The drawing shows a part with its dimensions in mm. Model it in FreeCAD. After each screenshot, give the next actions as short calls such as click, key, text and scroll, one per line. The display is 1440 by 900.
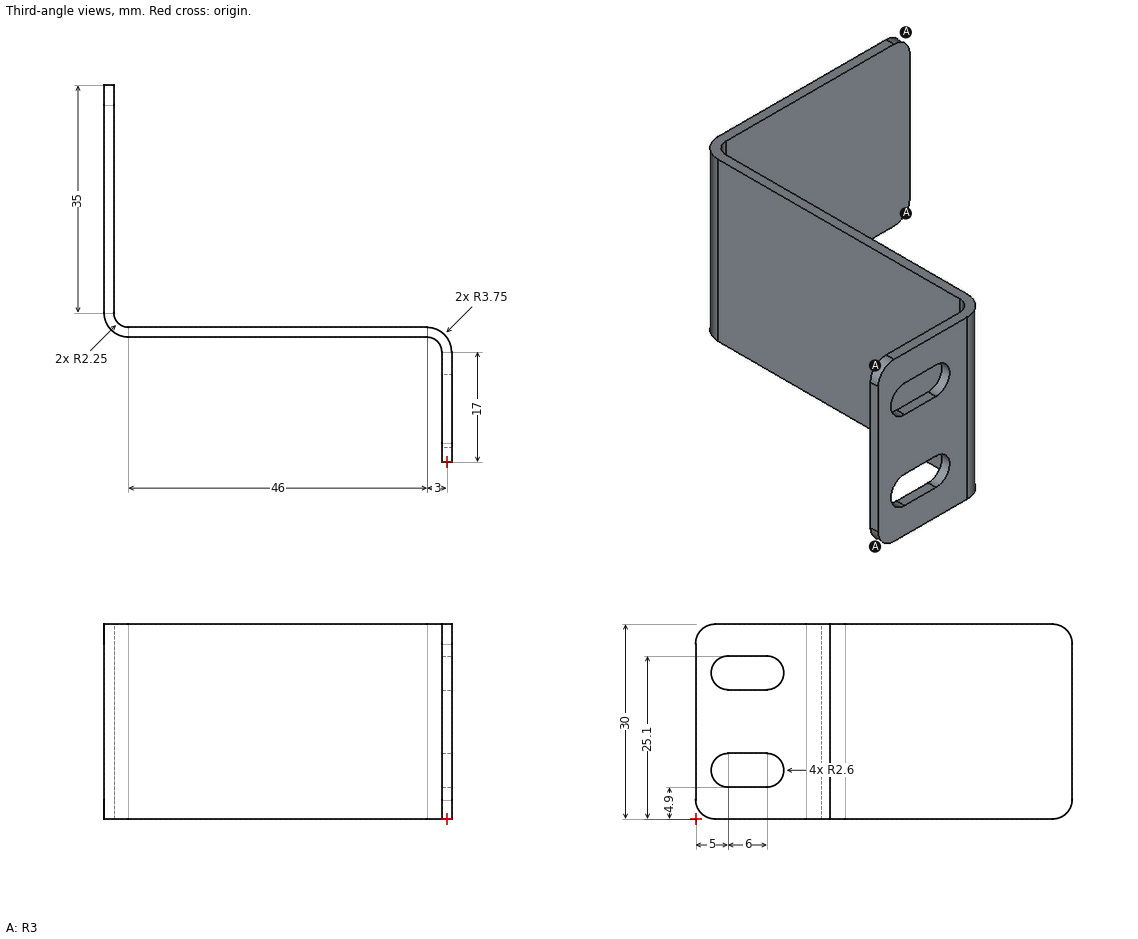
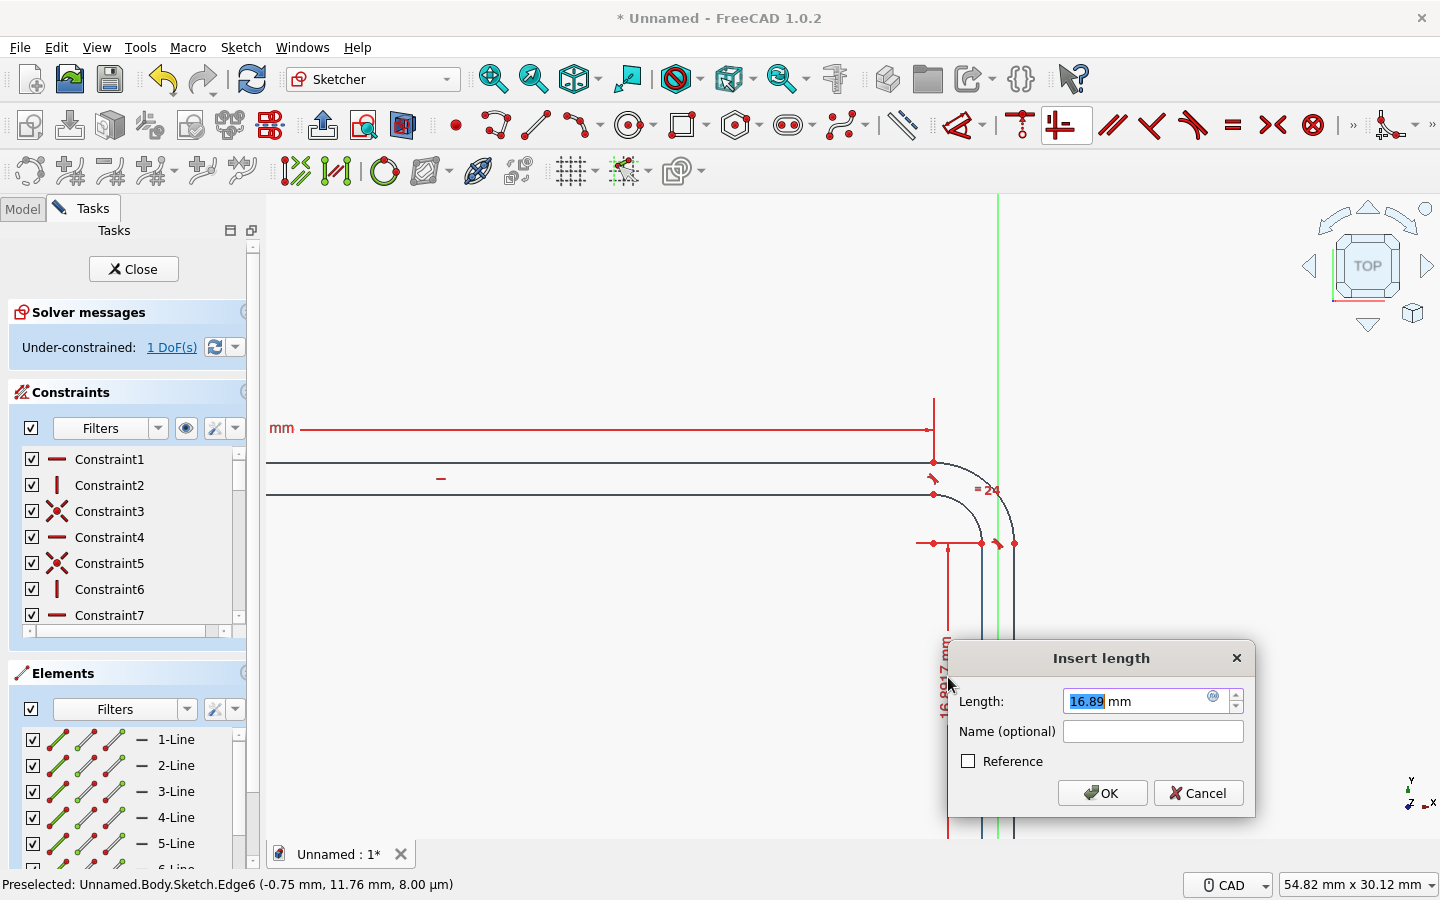
text(17)
key(Return)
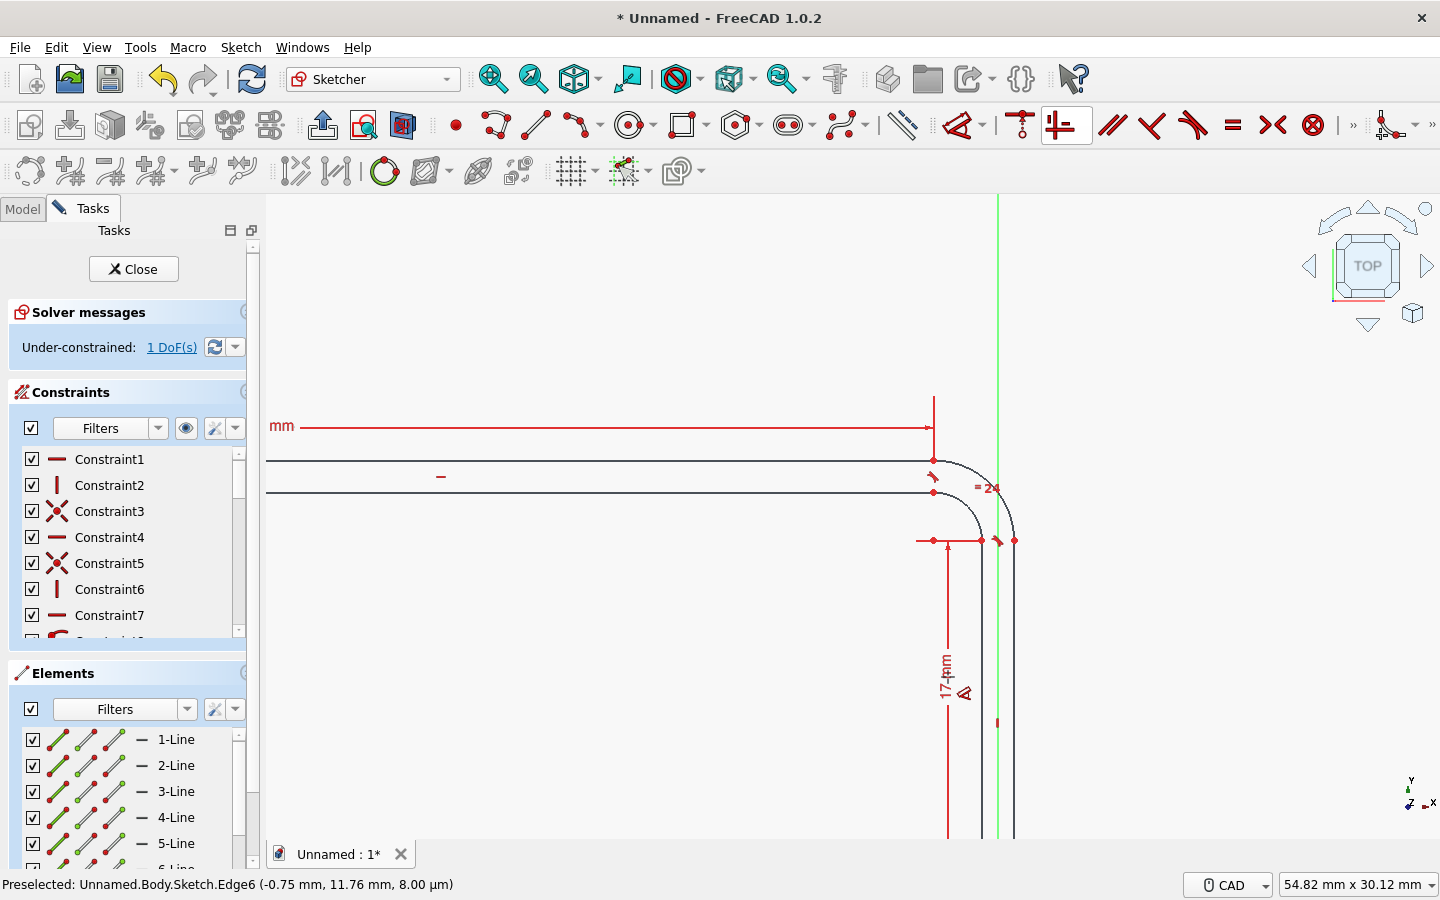
click(934, 461)
click(966, 427)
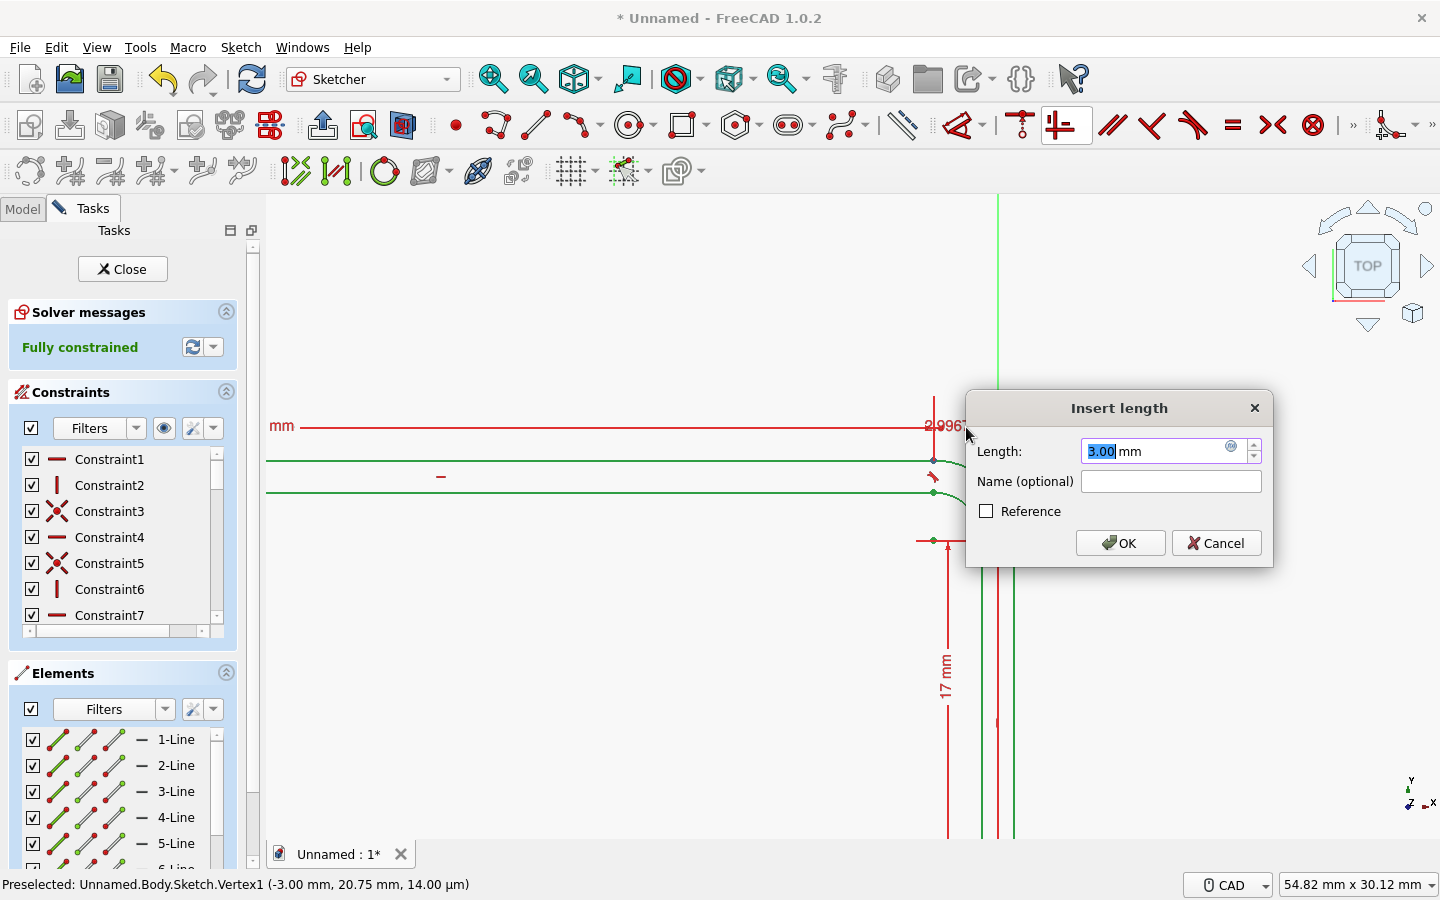
text(3)
key(Return)
key(Escape)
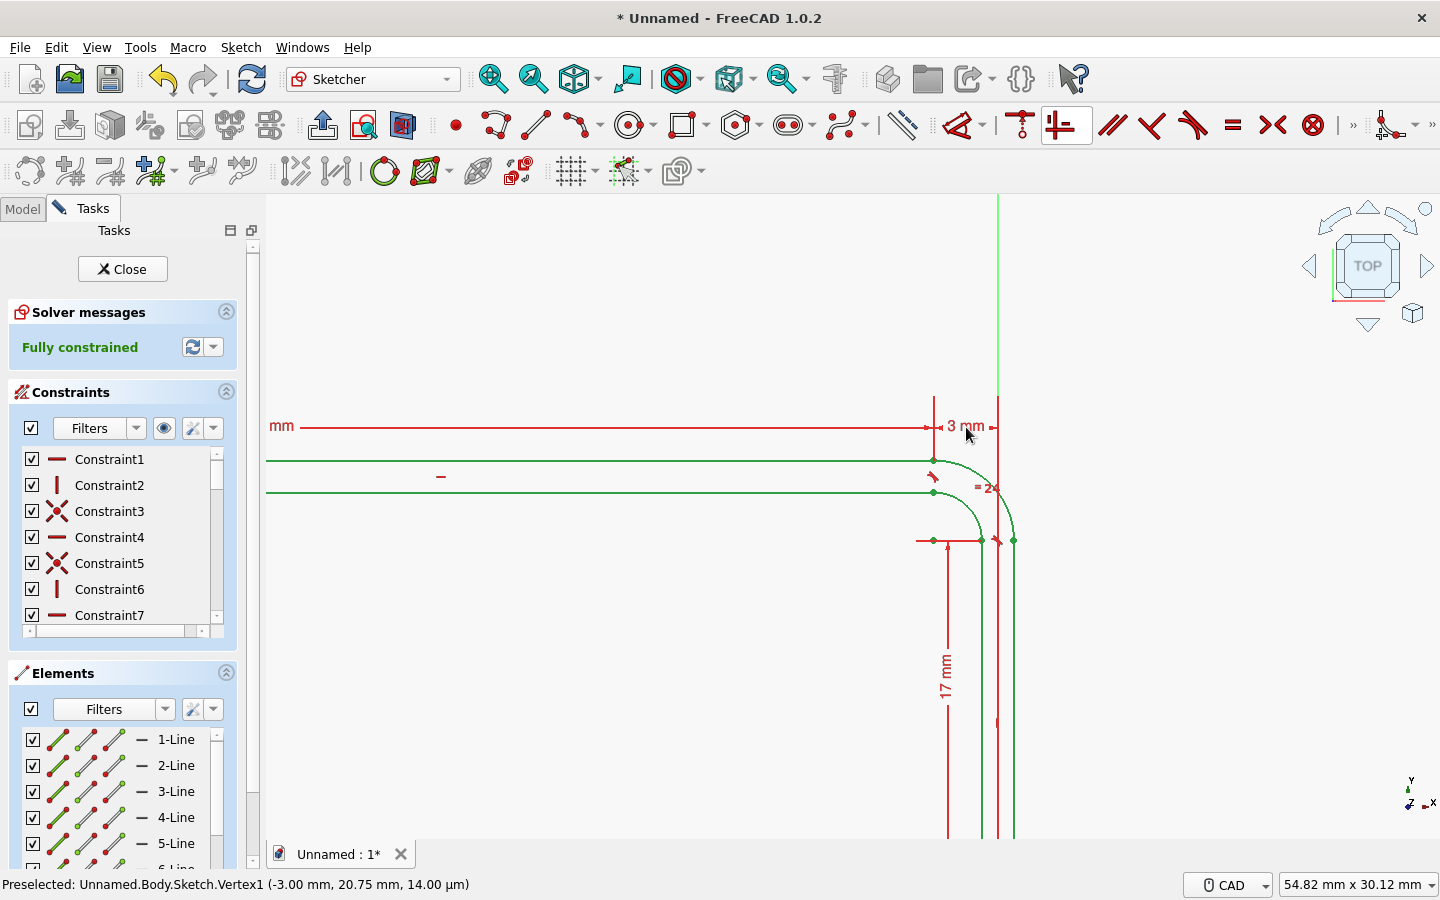
click(123, 269)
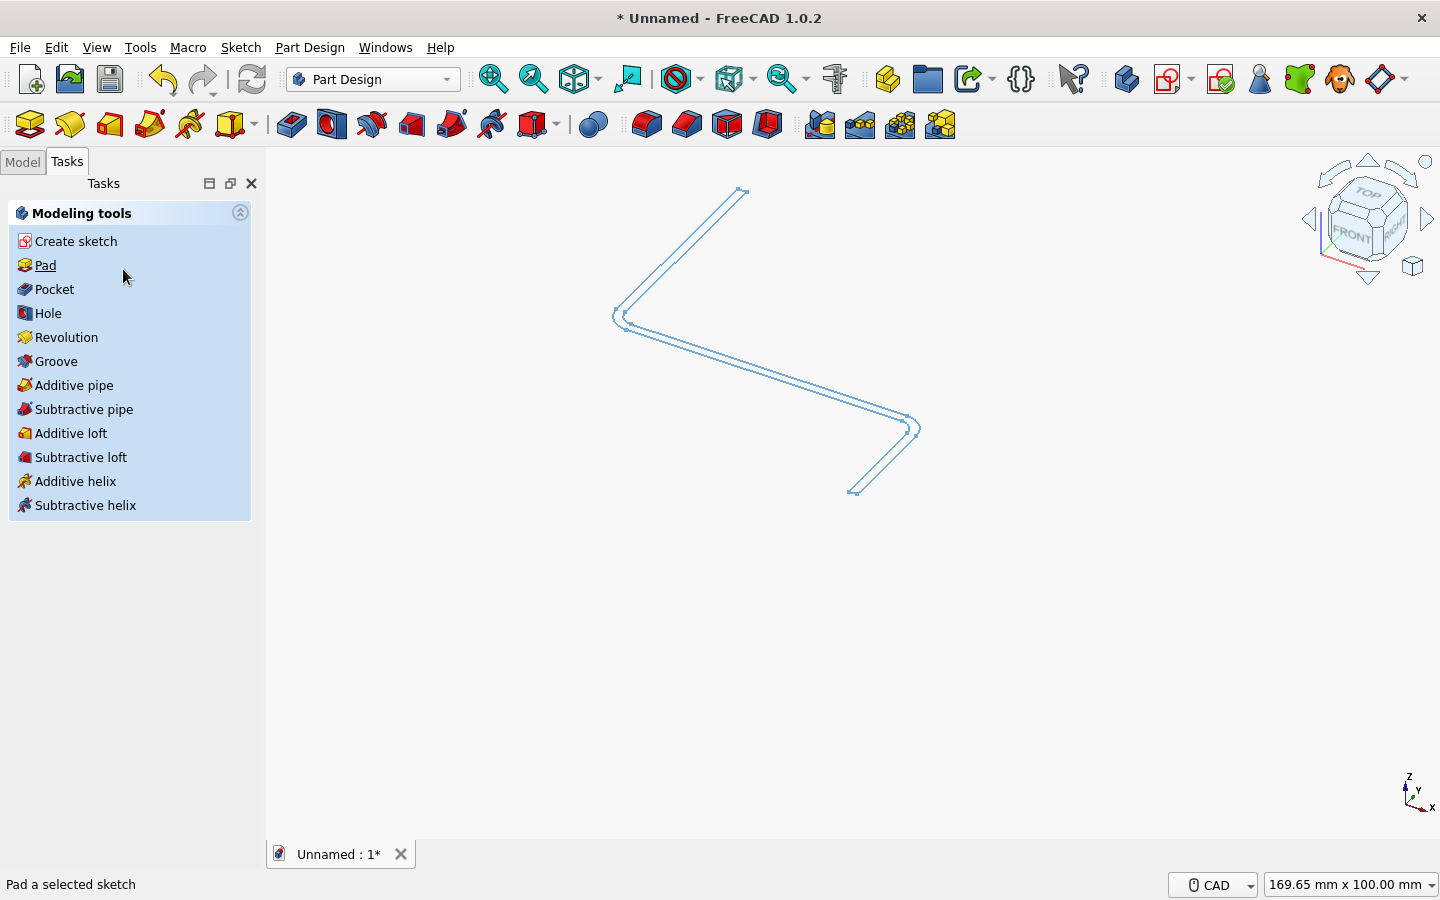
click(30, 124)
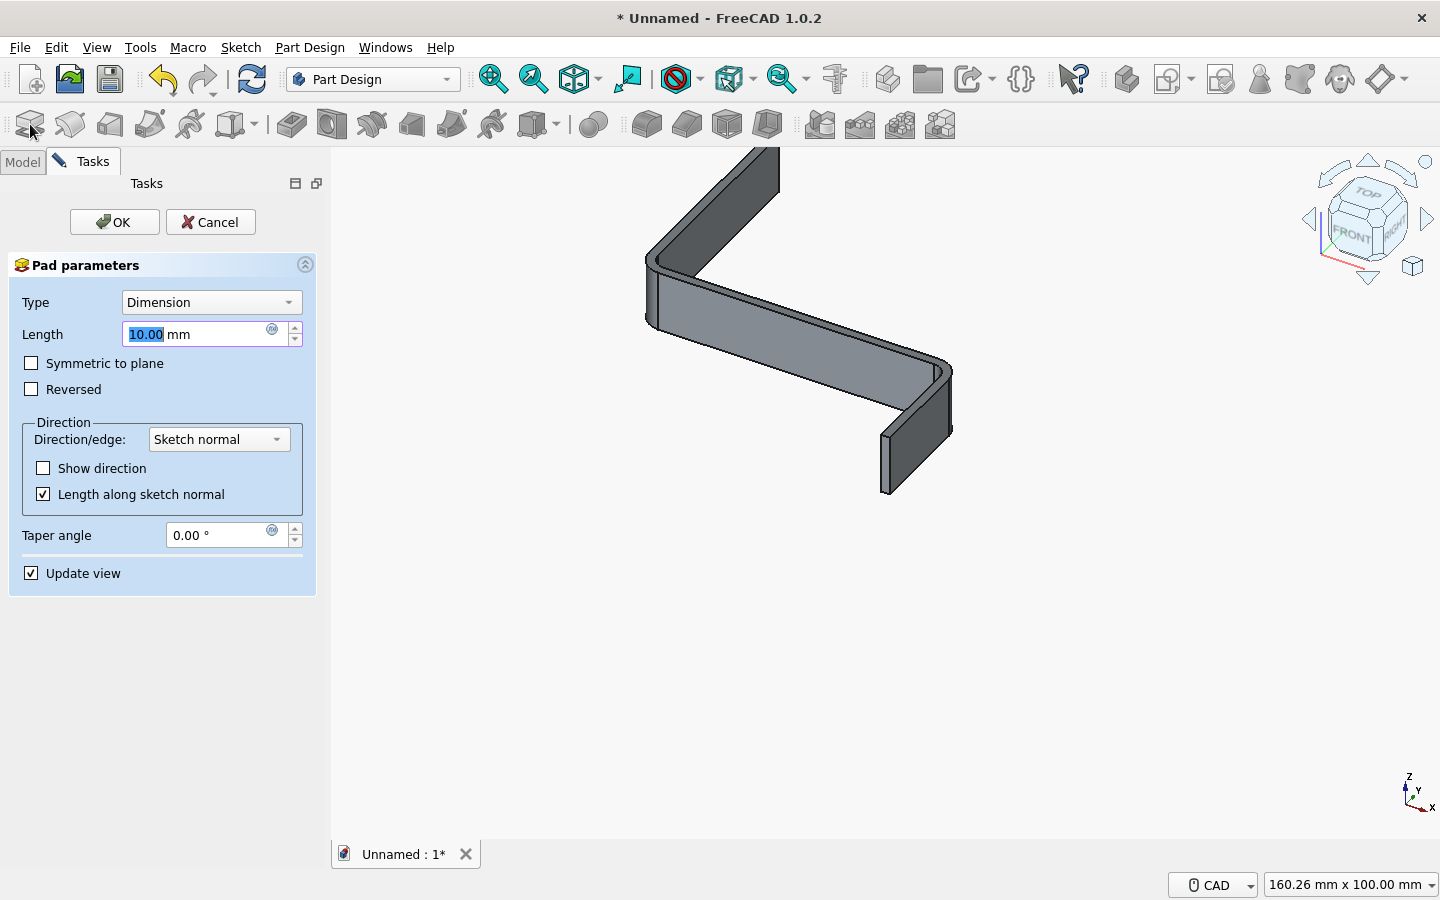
text(30)
key(Tab)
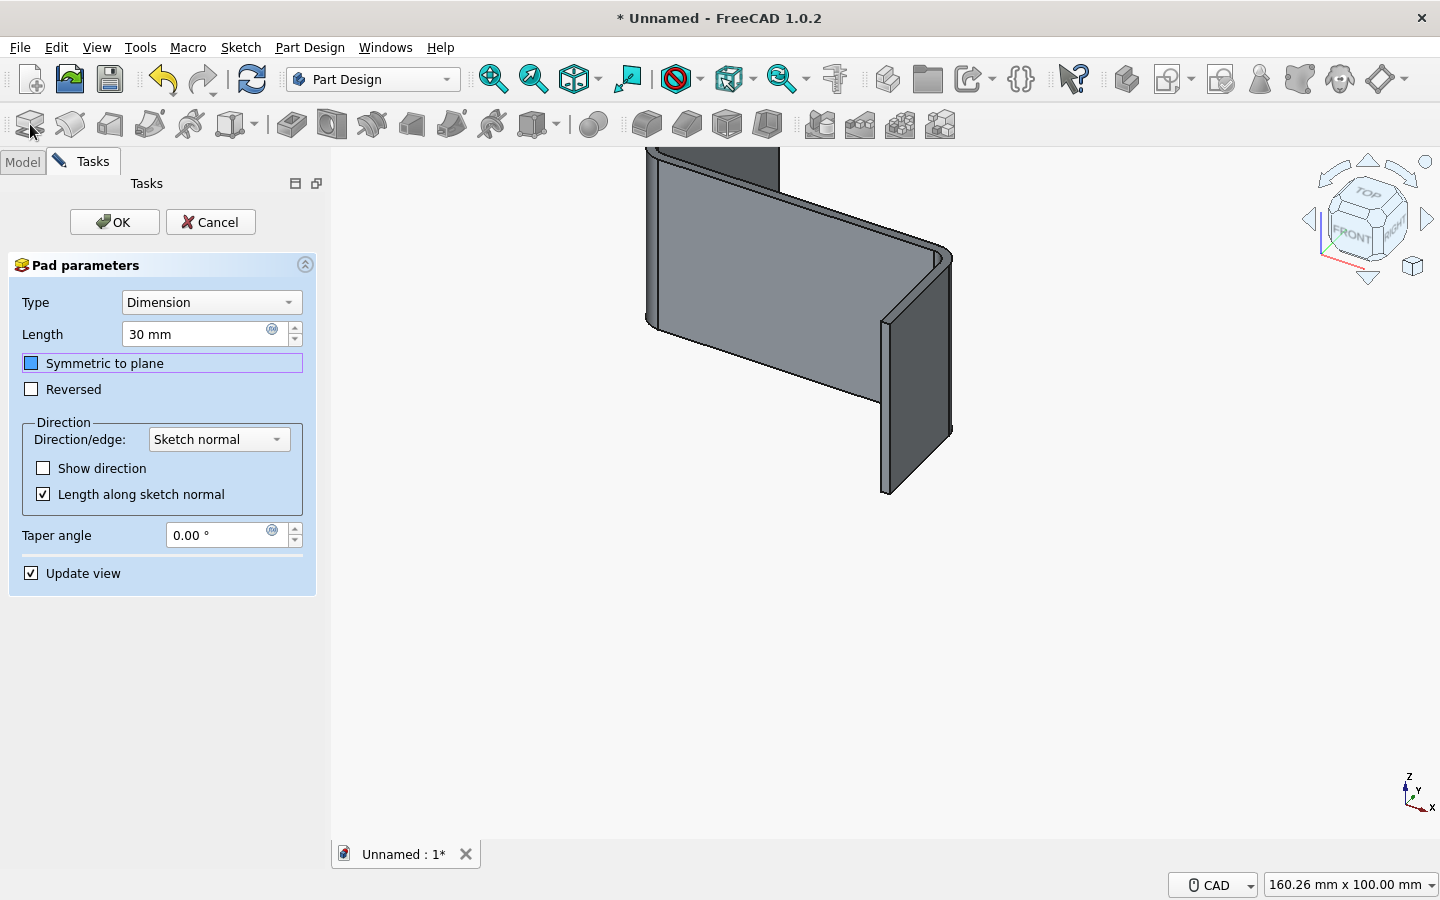
click(115, 222)